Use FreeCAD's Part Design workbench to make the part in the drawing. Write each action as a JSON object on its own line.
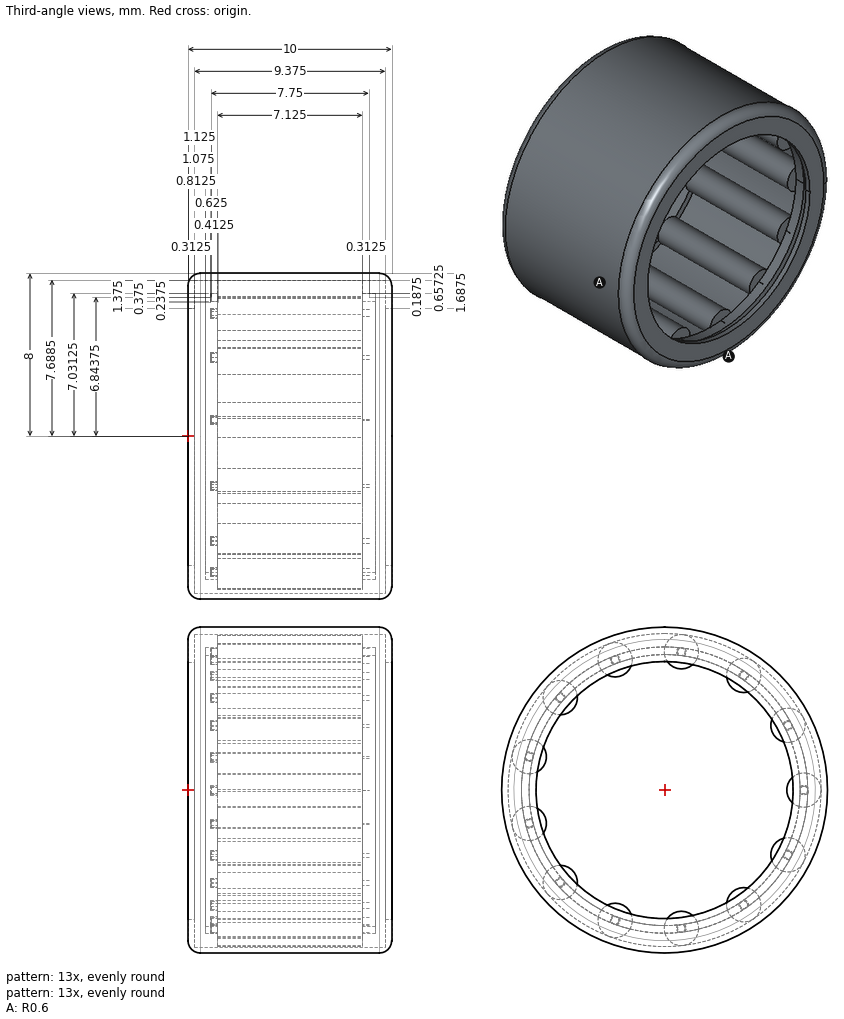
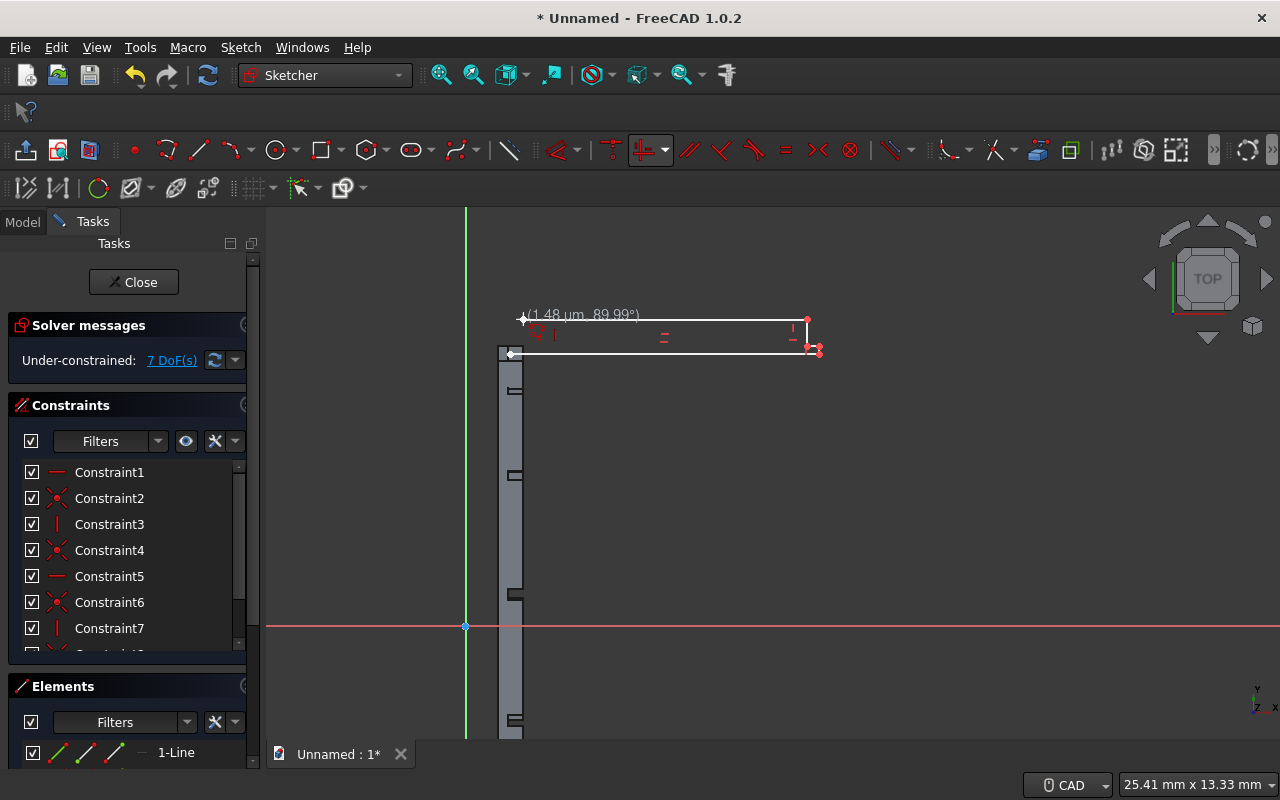
{"action": "scroll", "coordinate": [523, 346], "scroll_direction": "up", "scroll_amount": 4}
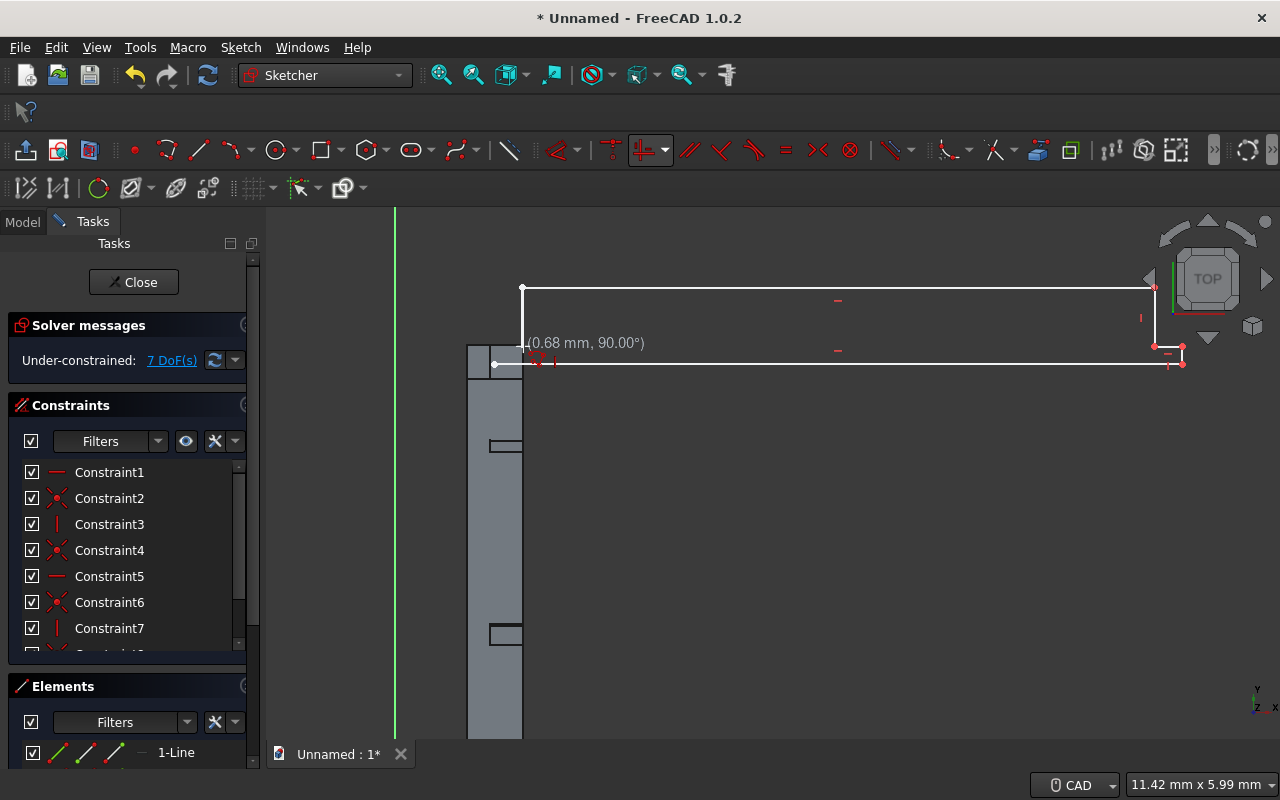
{"action": "left_click", "coordinate": [523, 345]}
{"action": "left_click", "coordinate": [495, 345]}
{"action": "left_click", "coordinate": [494, 364]}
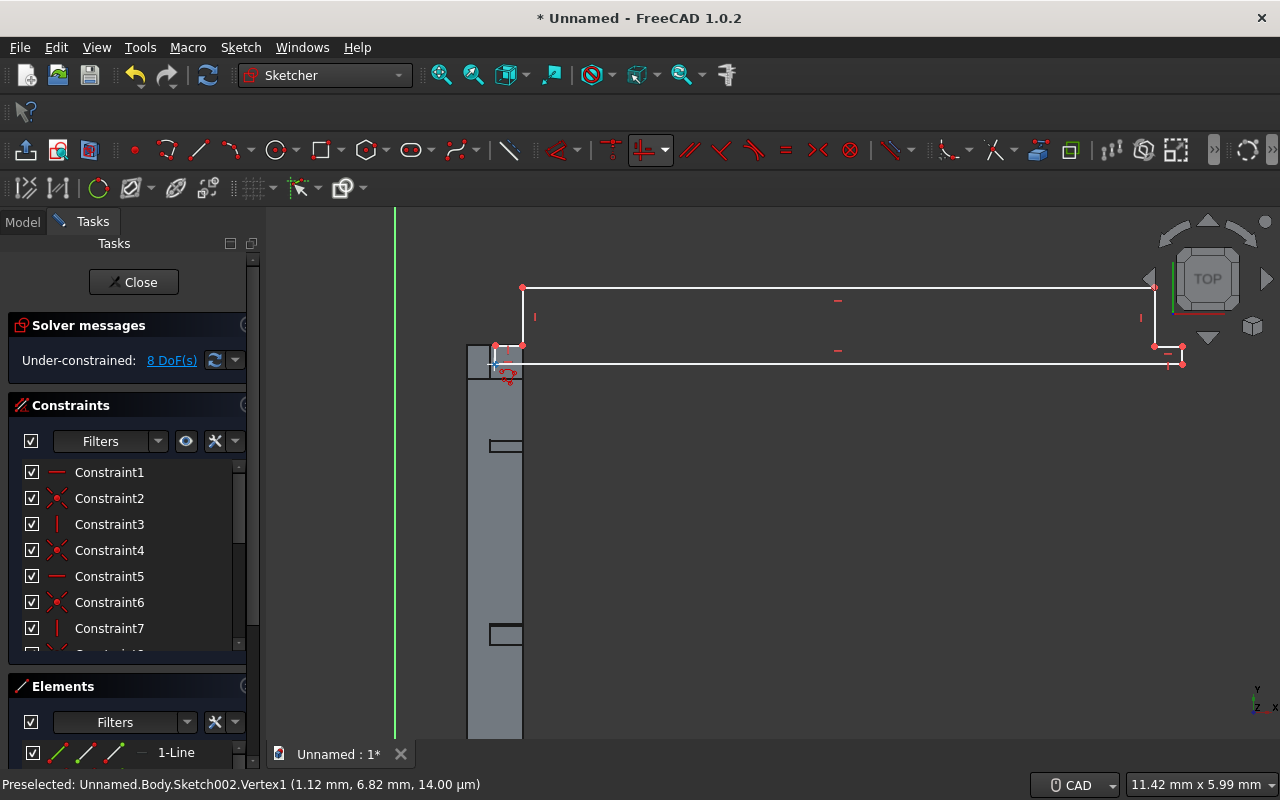
{"action": "left_click", "coordinate": [200, 150]}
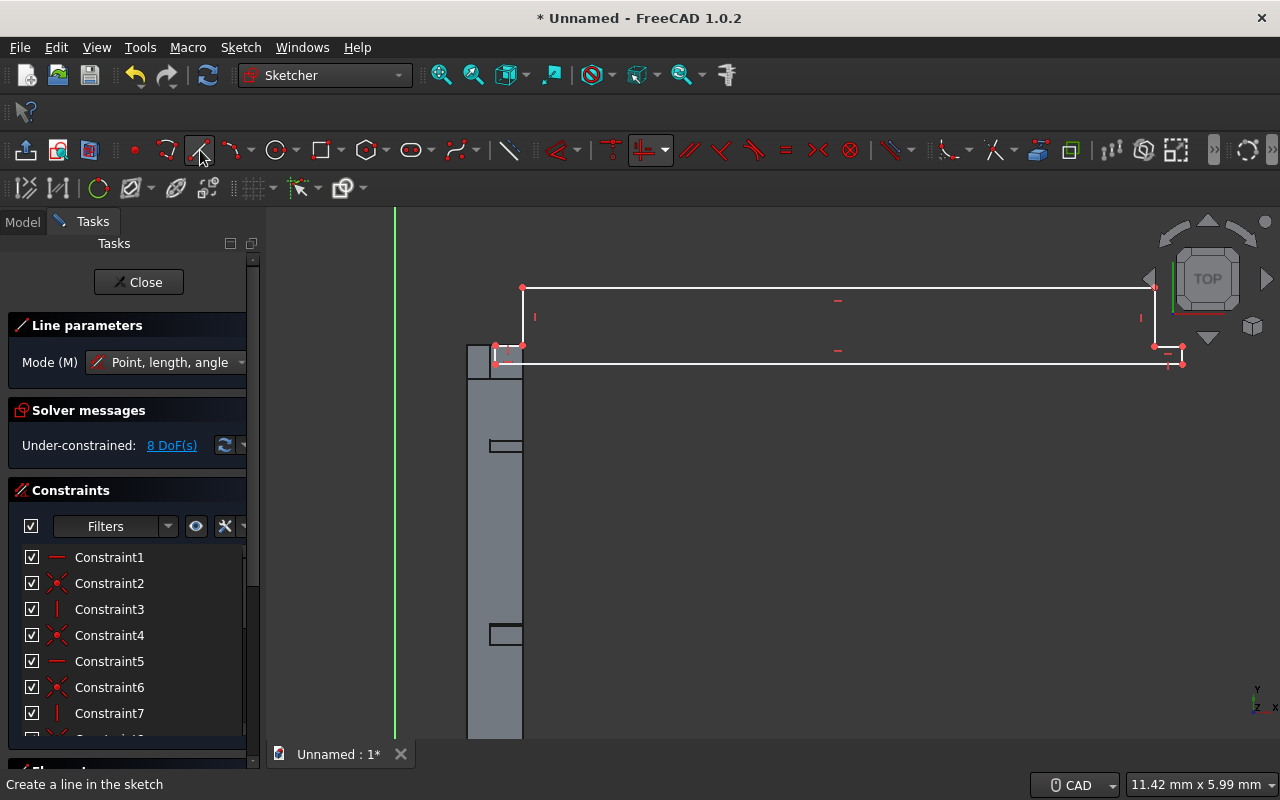
{"action": "scroll", "coordinate": [523, 346], "scroll_direction": "down", "scroll_amount": 4}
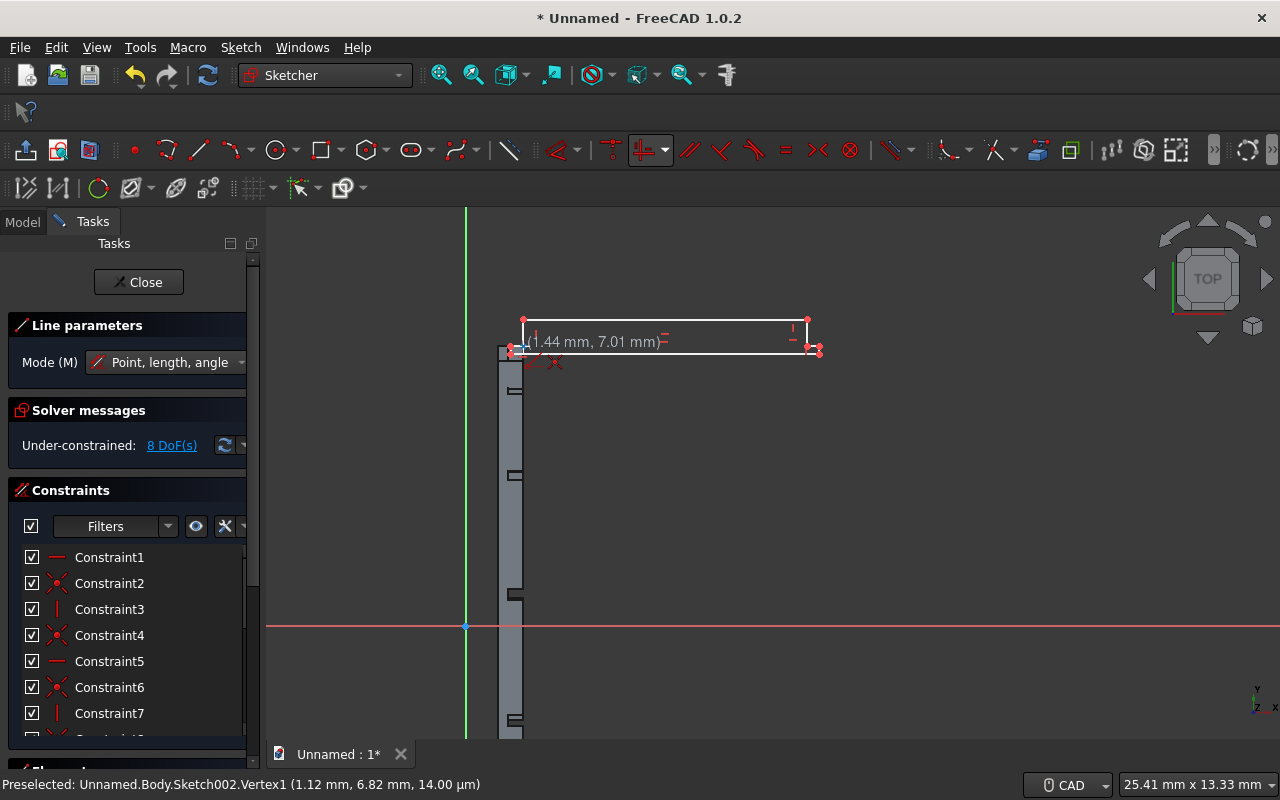
{"action": "left_click", "coordinate": [851, 353]}
{"action": "left_click", "coordinate": [943, 353]}
{"action": "key", "text": "Escape"}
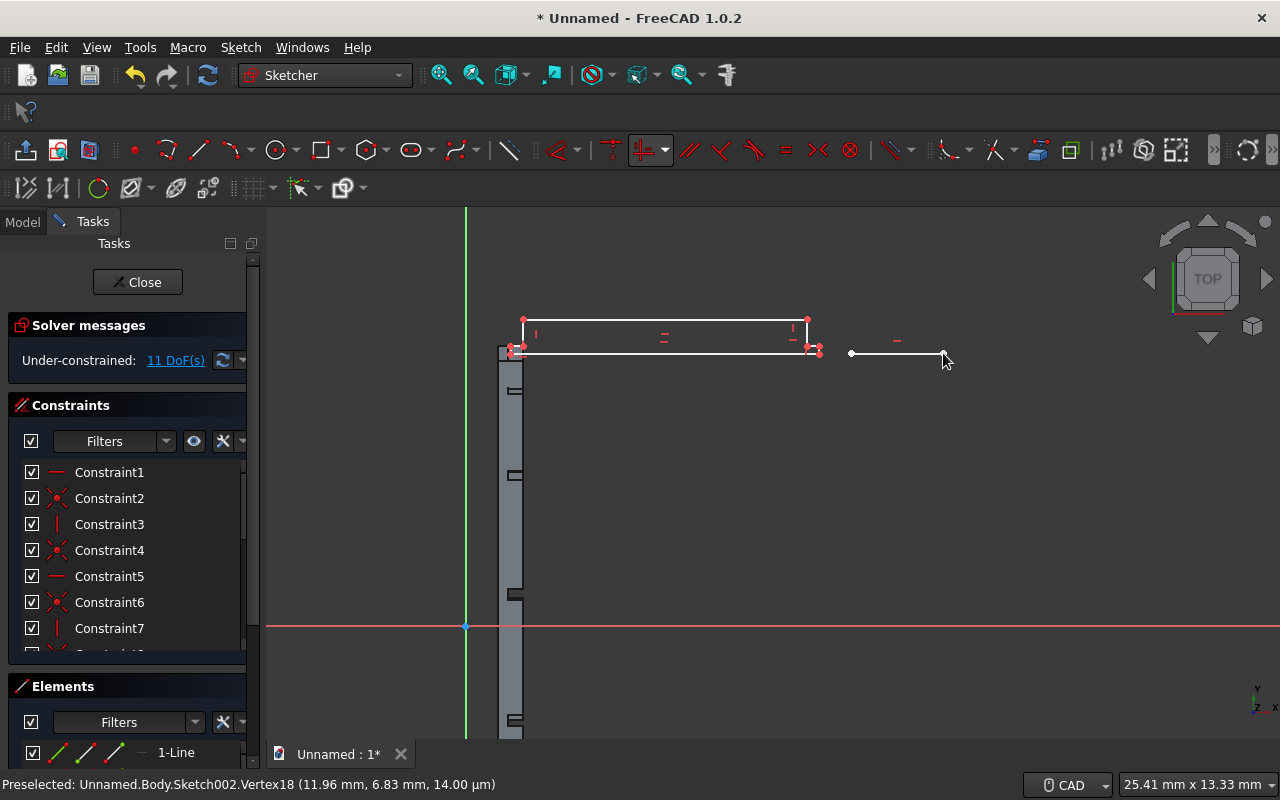
{"action": "left_click", "coordinate": [879, 354]}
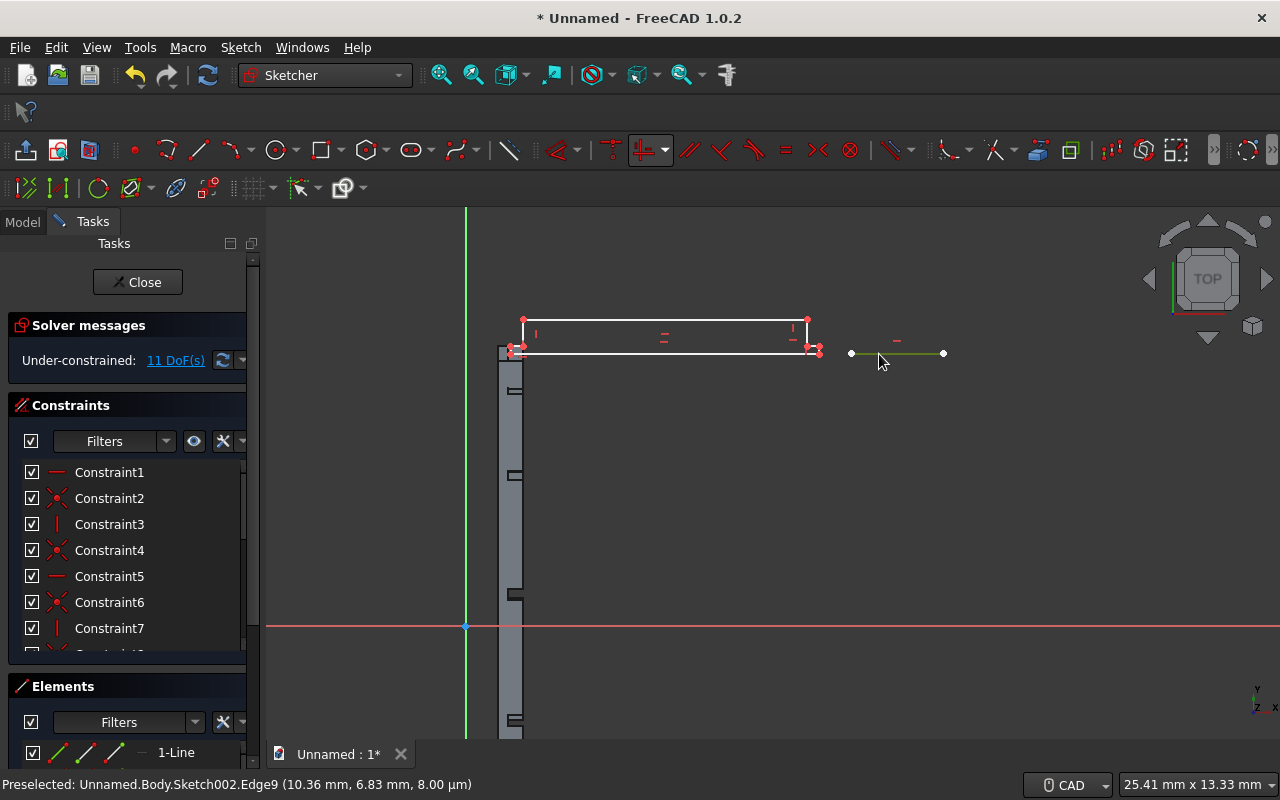
{"action": "left_click", "coordinate": [510, 150]}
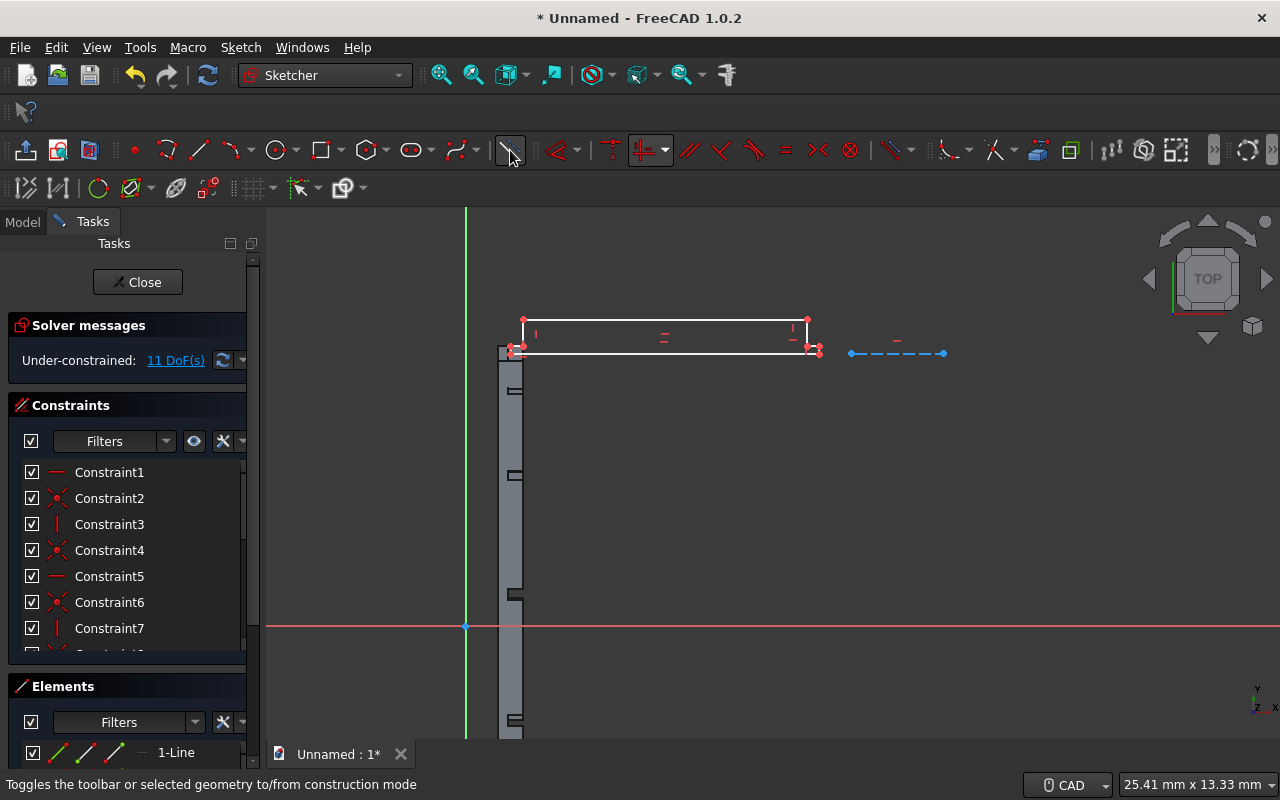
{"action": "left_click", "coordinate": [556, 150]}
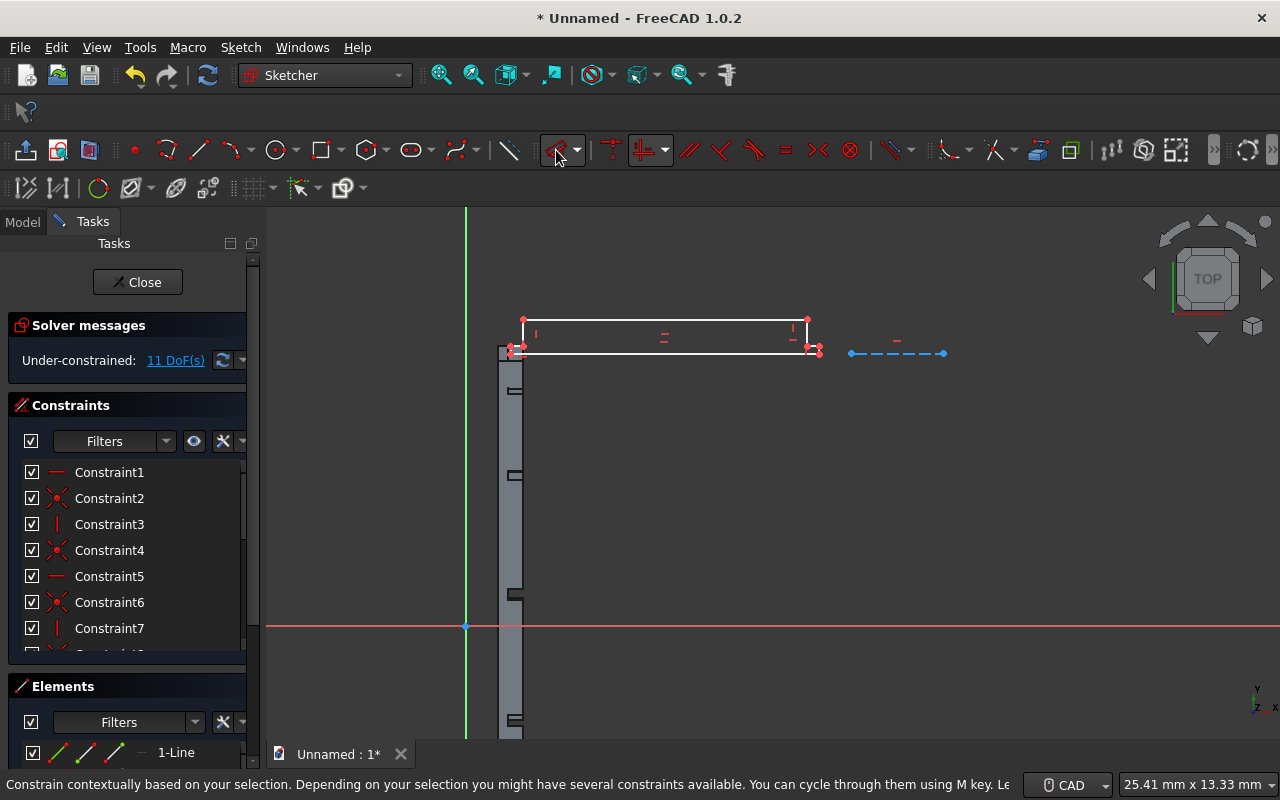
{"action": "left_click", "coordinate": [603, 354]}
{"action": "left_click", "coordinate": [665, 388]}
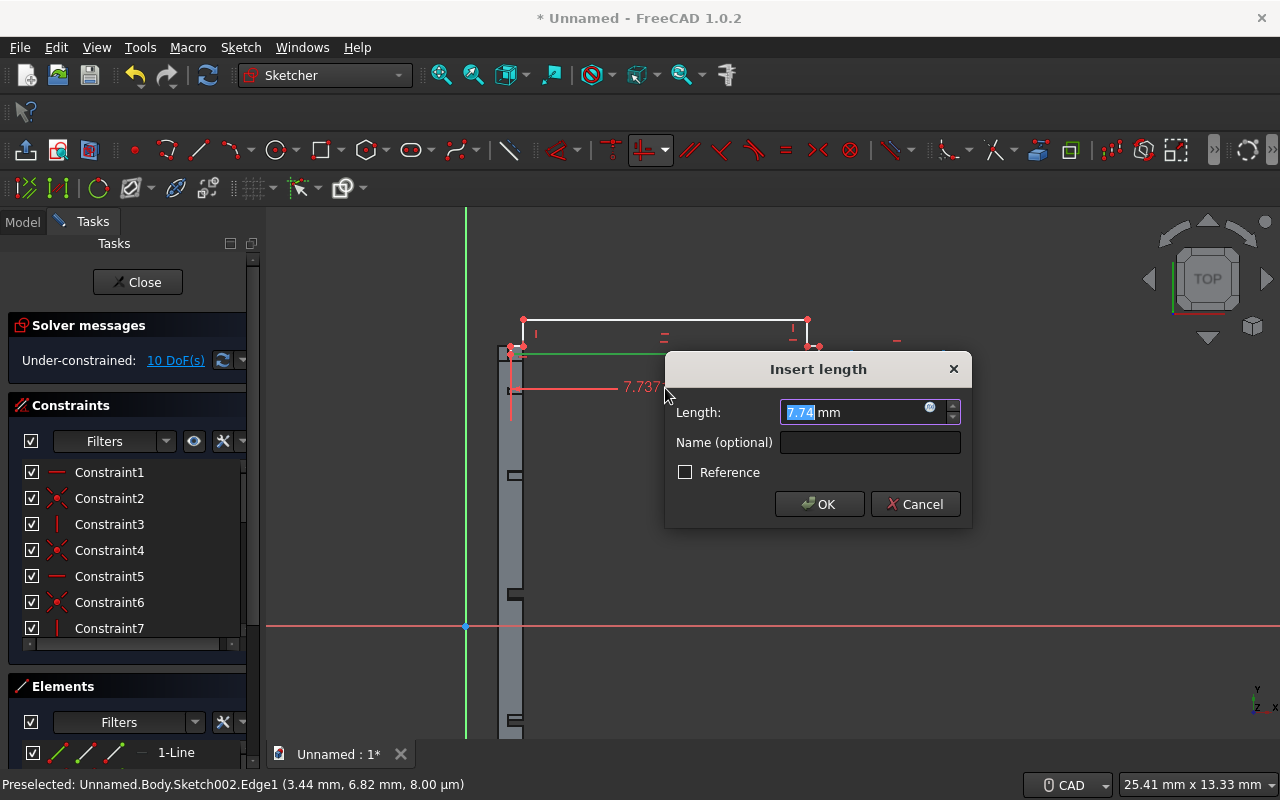
{"action": "type", "text": "7.75"}
{"action": "key", "text": "Return"}